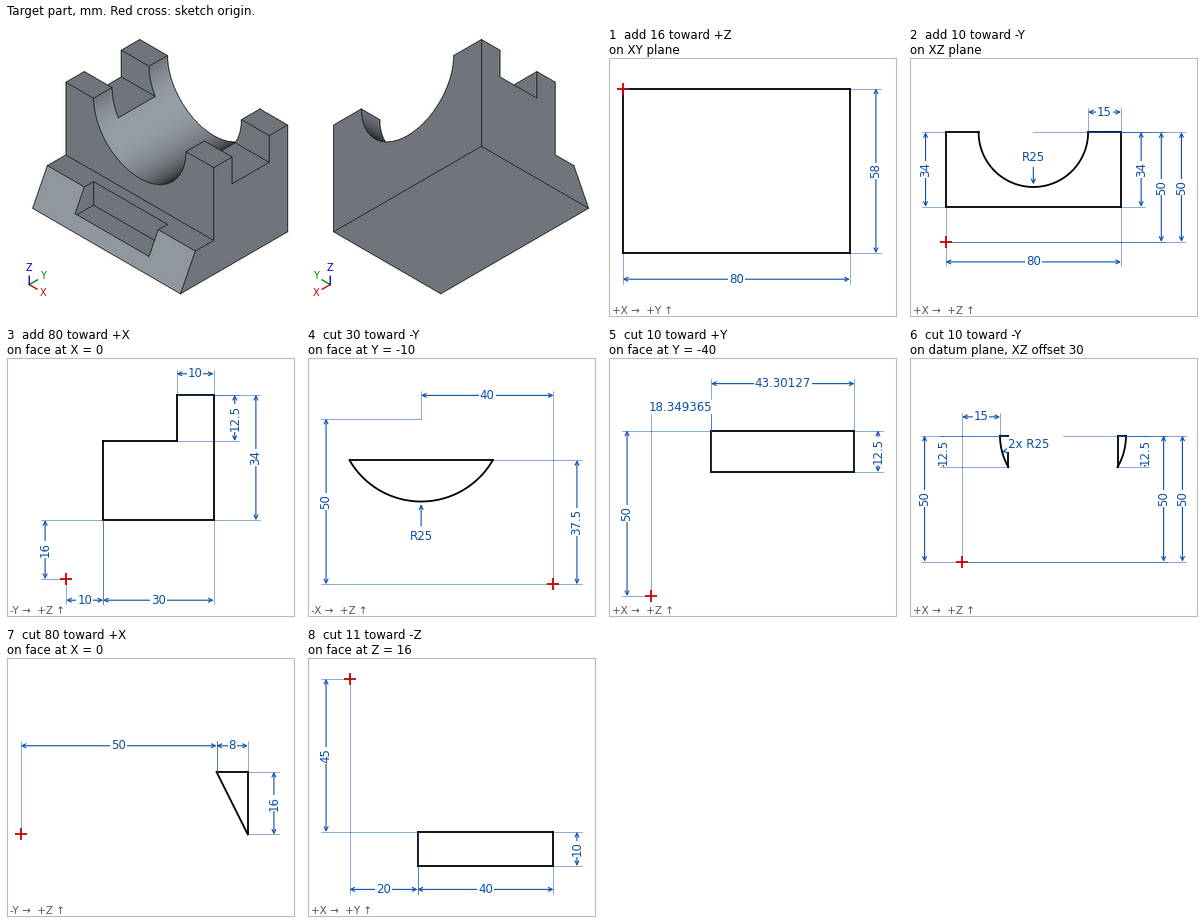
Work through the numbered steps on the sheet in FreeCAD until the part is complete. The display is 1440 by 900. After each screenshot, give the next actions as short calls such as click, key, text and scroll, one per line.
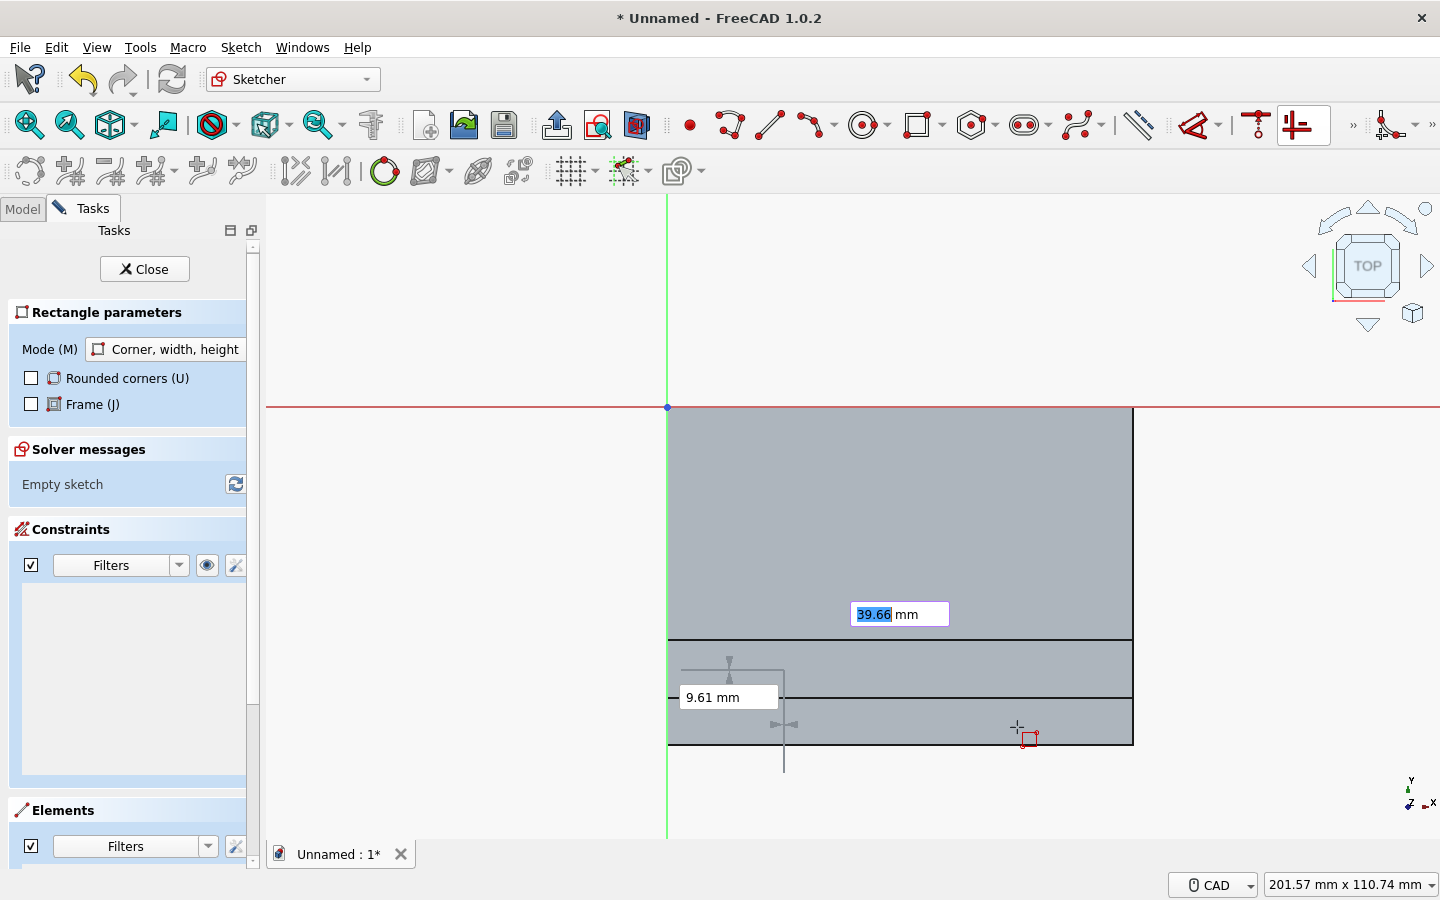
text(40)
key(Tab)
text(10)
key(Return)
key(Escape)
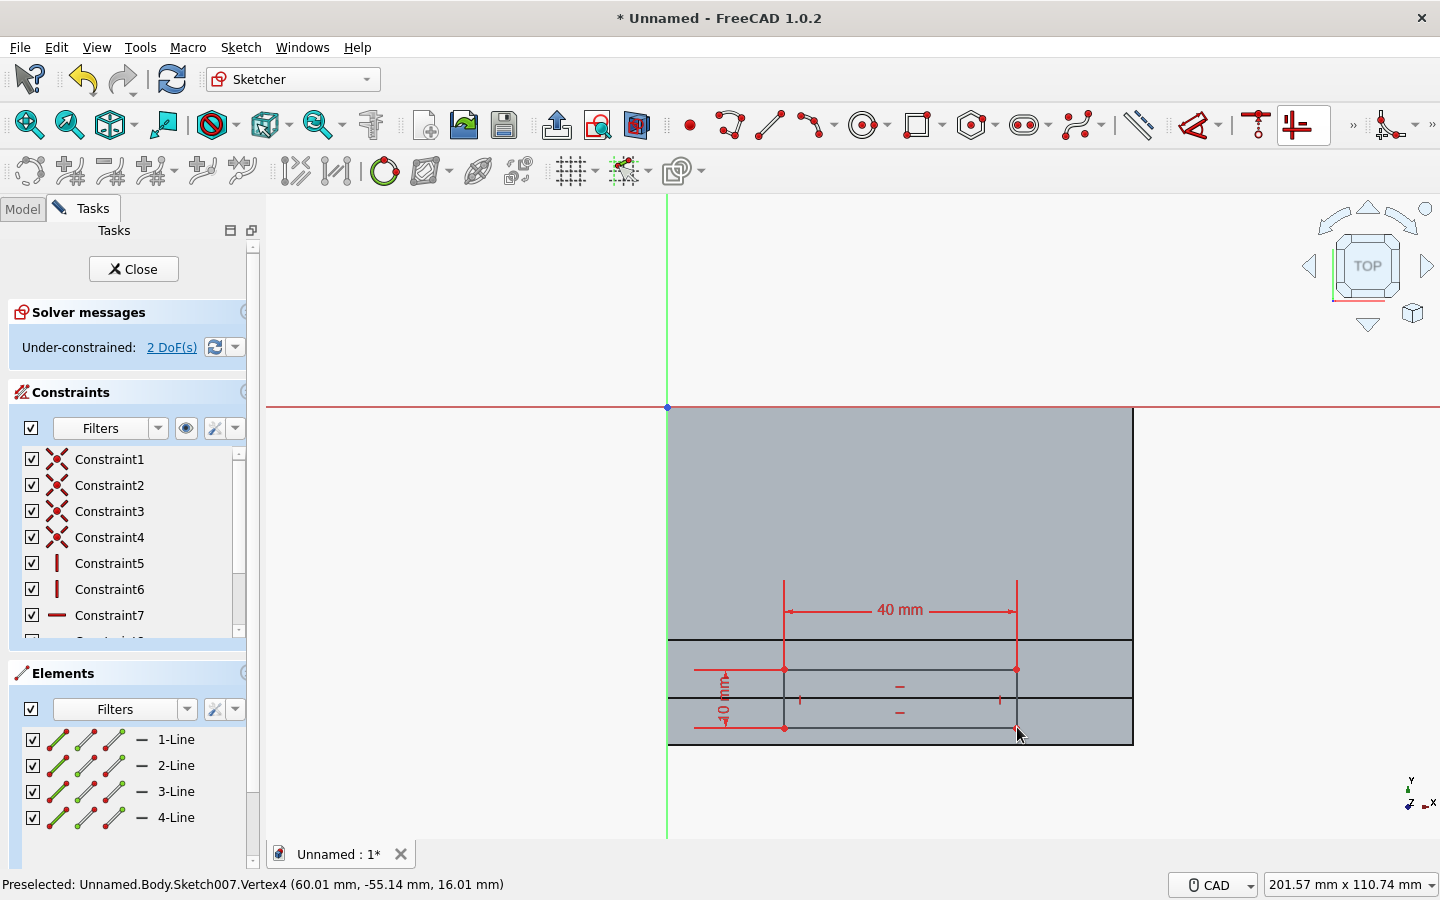
click(1194, 126)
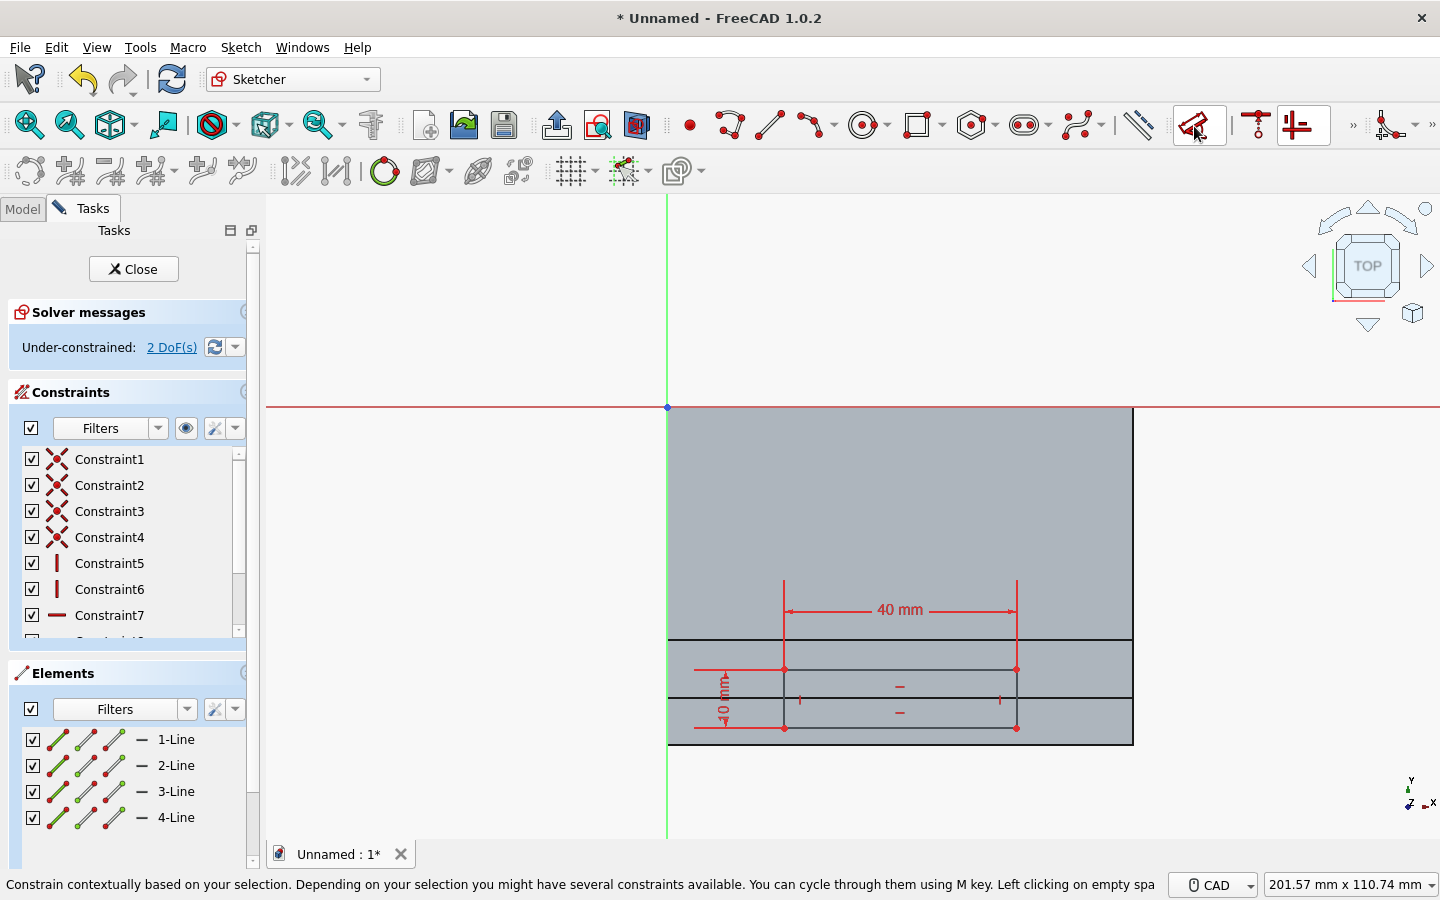
click(784, 670)
click(726, 373)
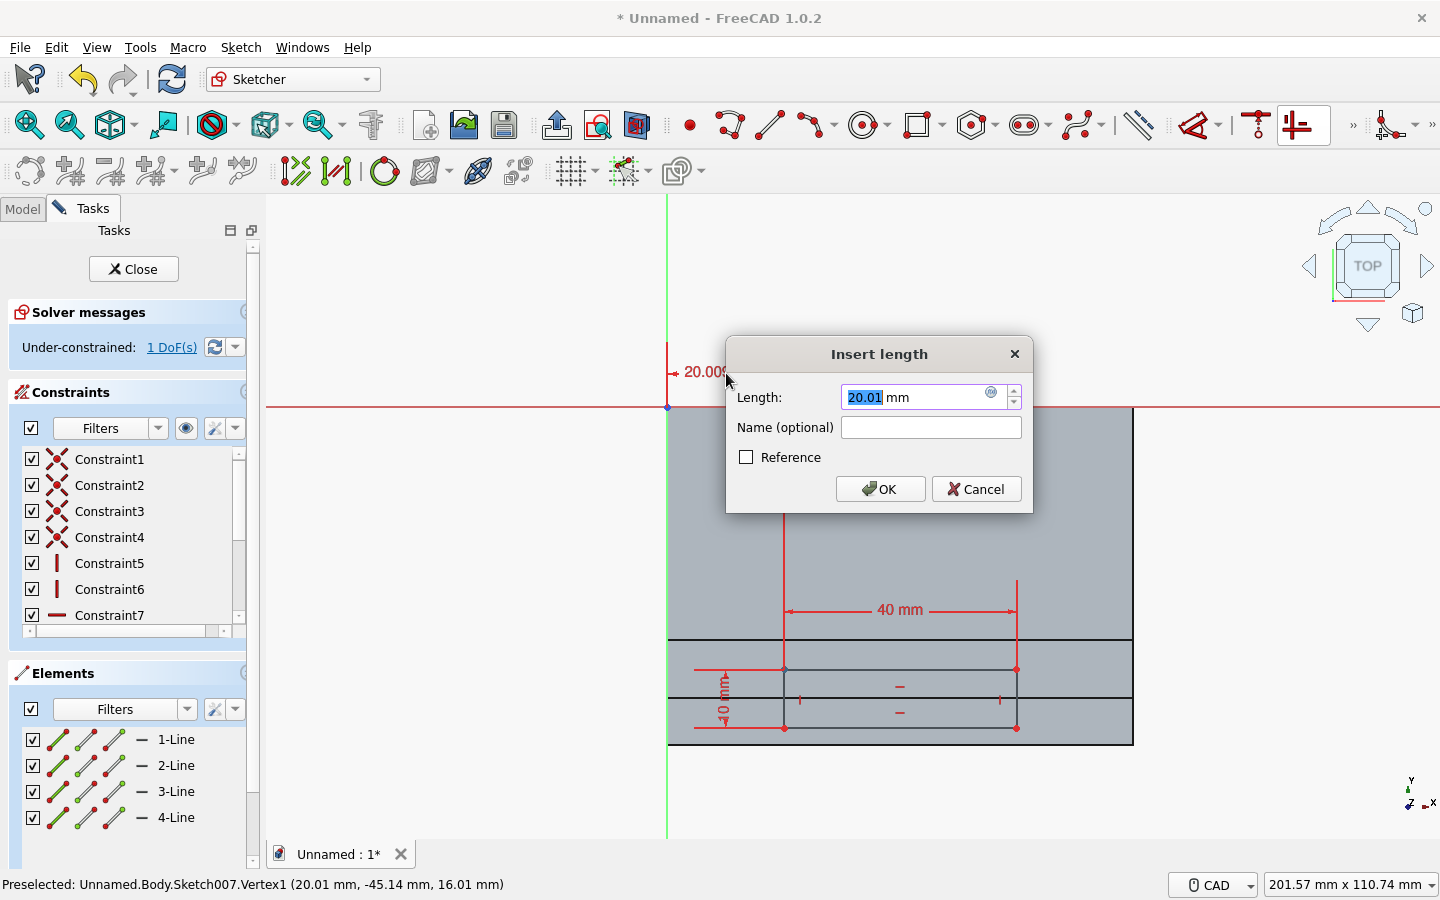
text(20)
key(Return)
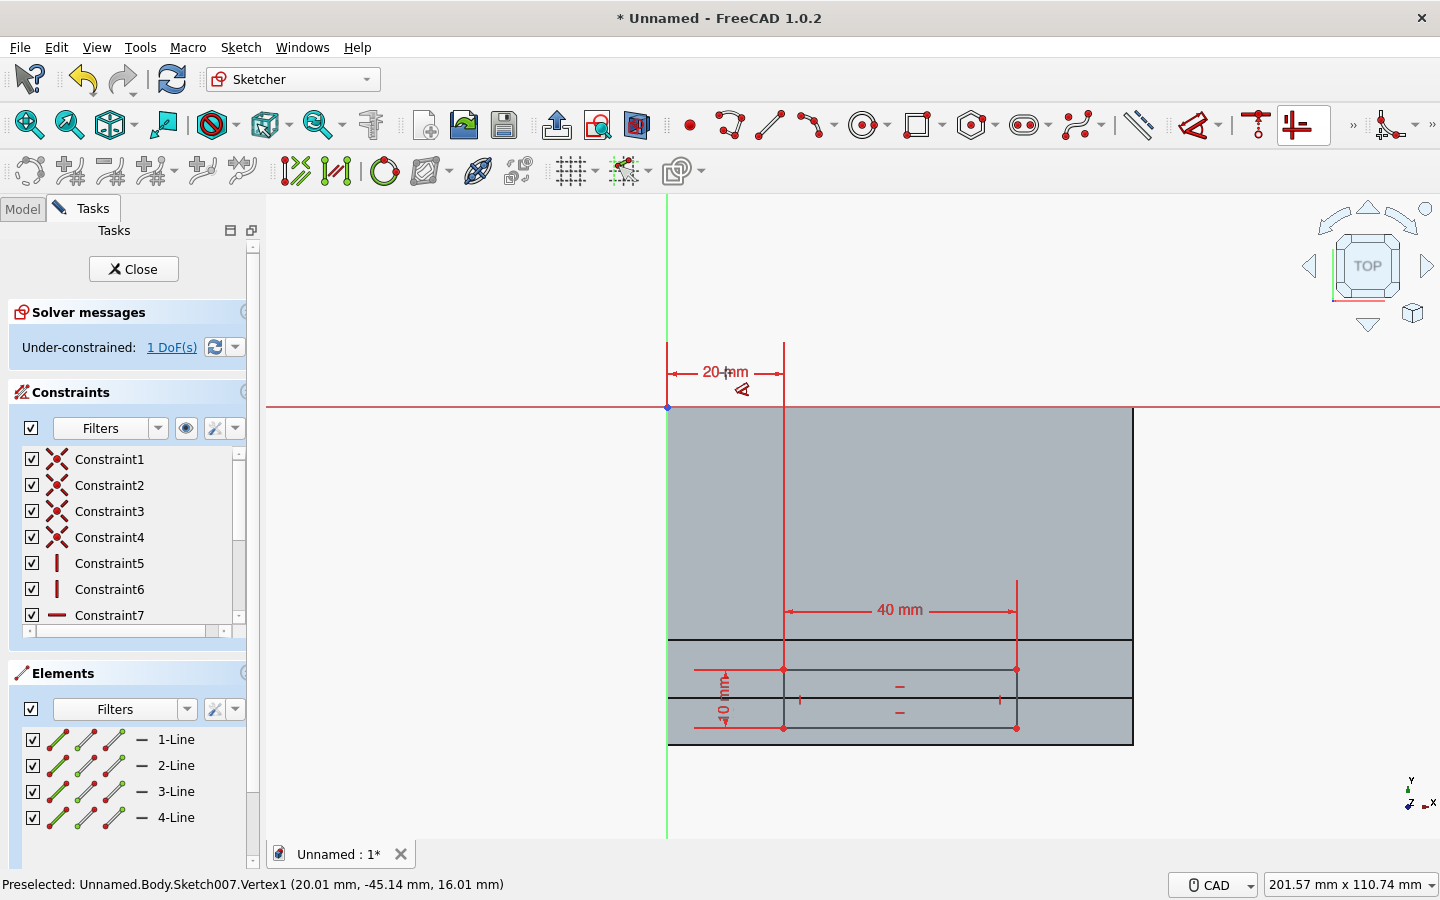
click(784, 670)
click(633, 539)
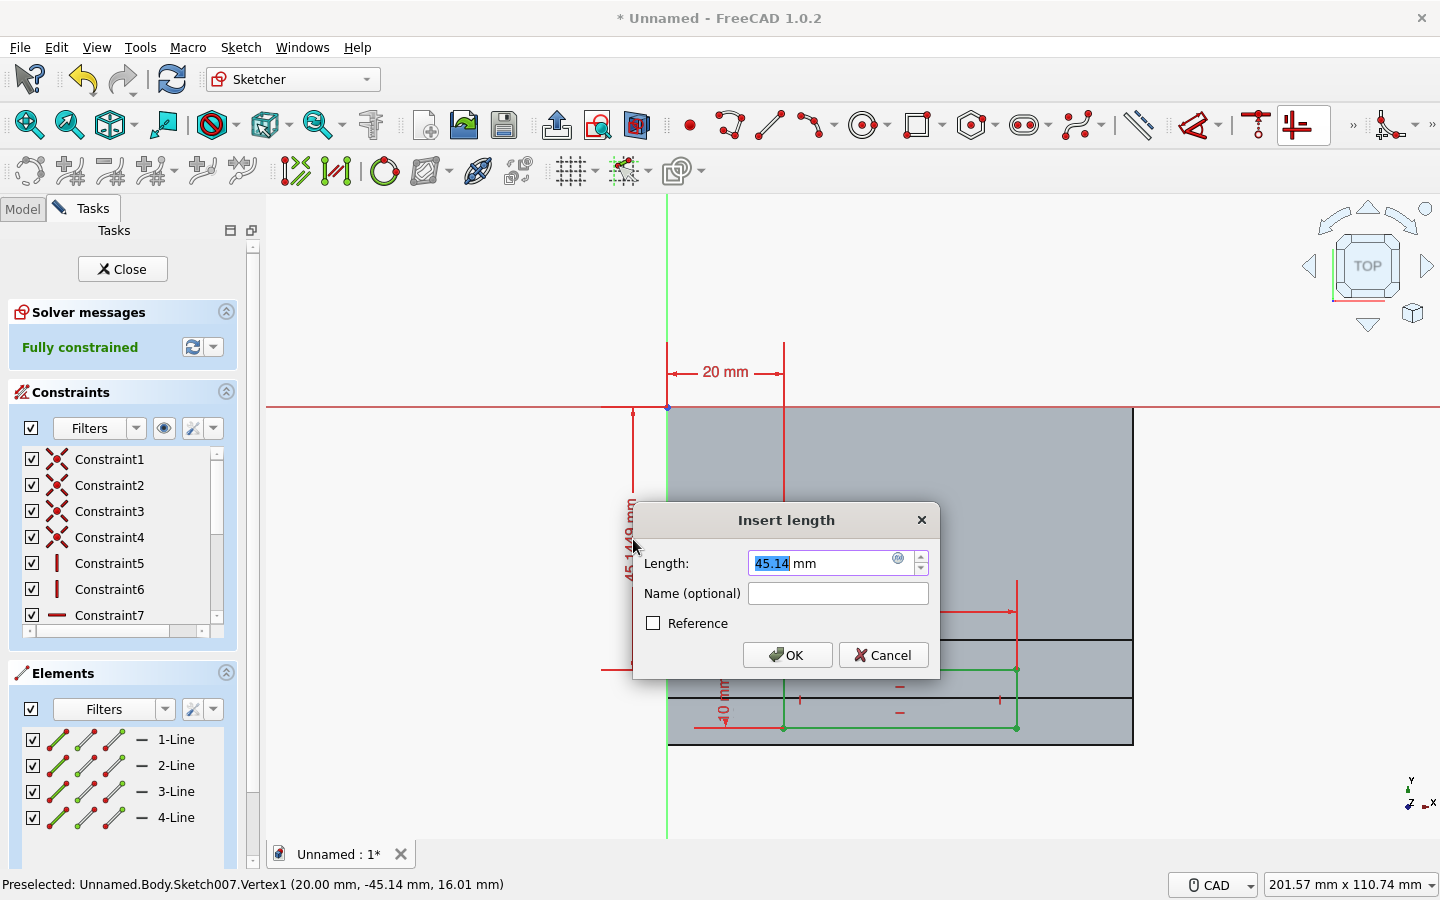
text(45)
key(Return)
key(Escape)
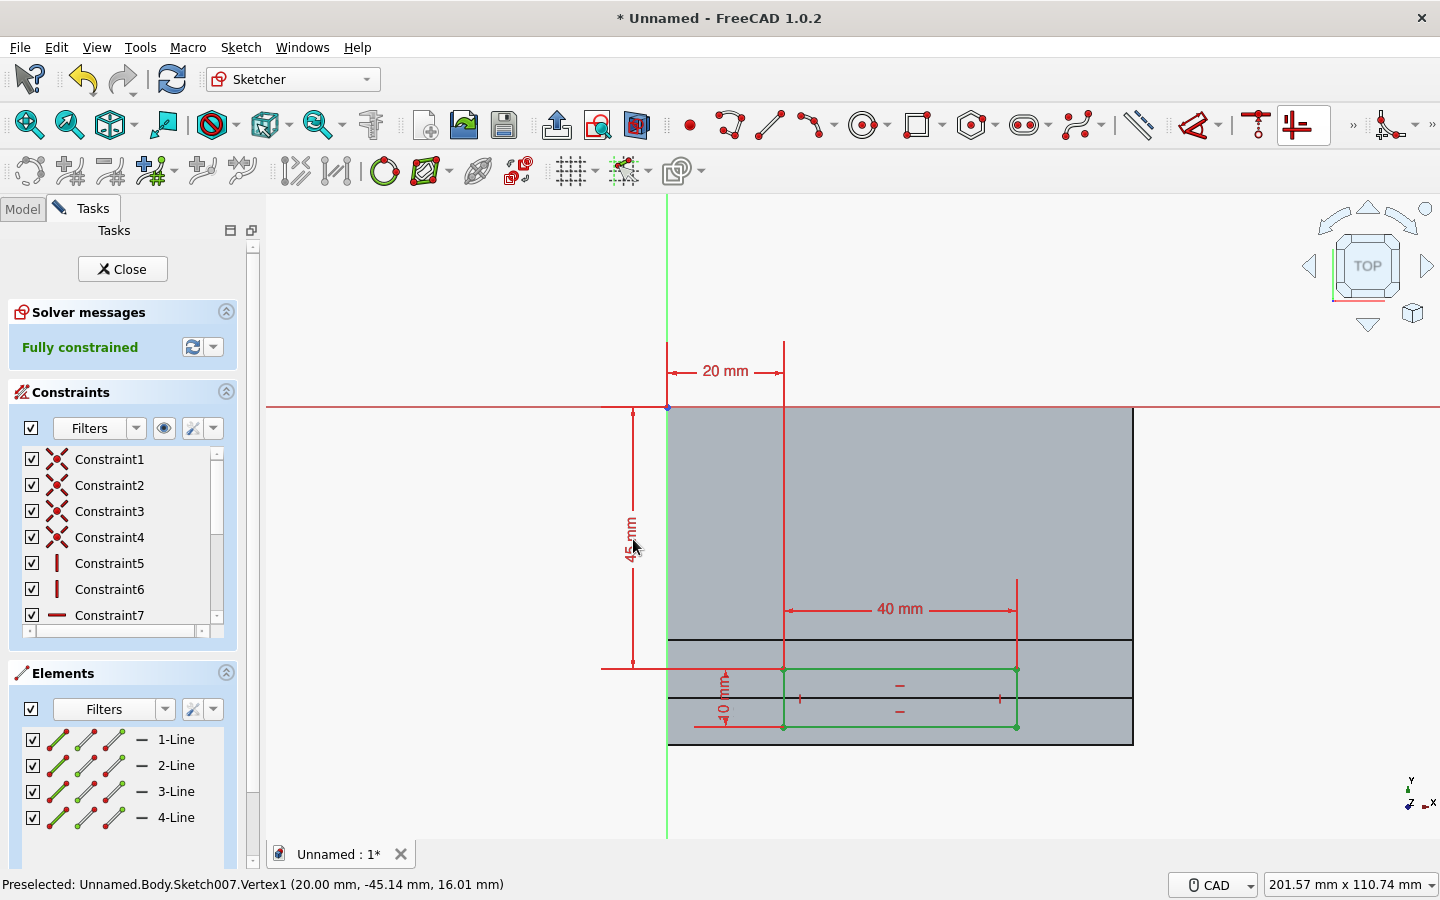
click(123, 269)